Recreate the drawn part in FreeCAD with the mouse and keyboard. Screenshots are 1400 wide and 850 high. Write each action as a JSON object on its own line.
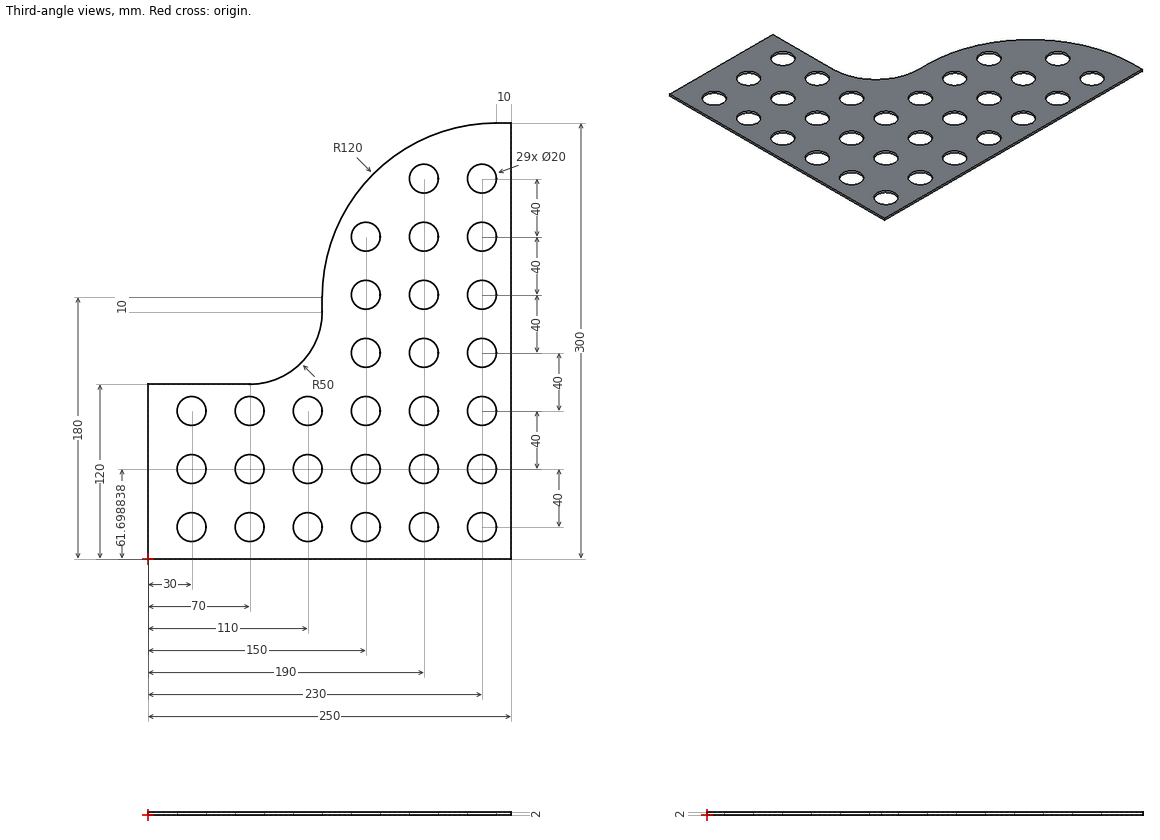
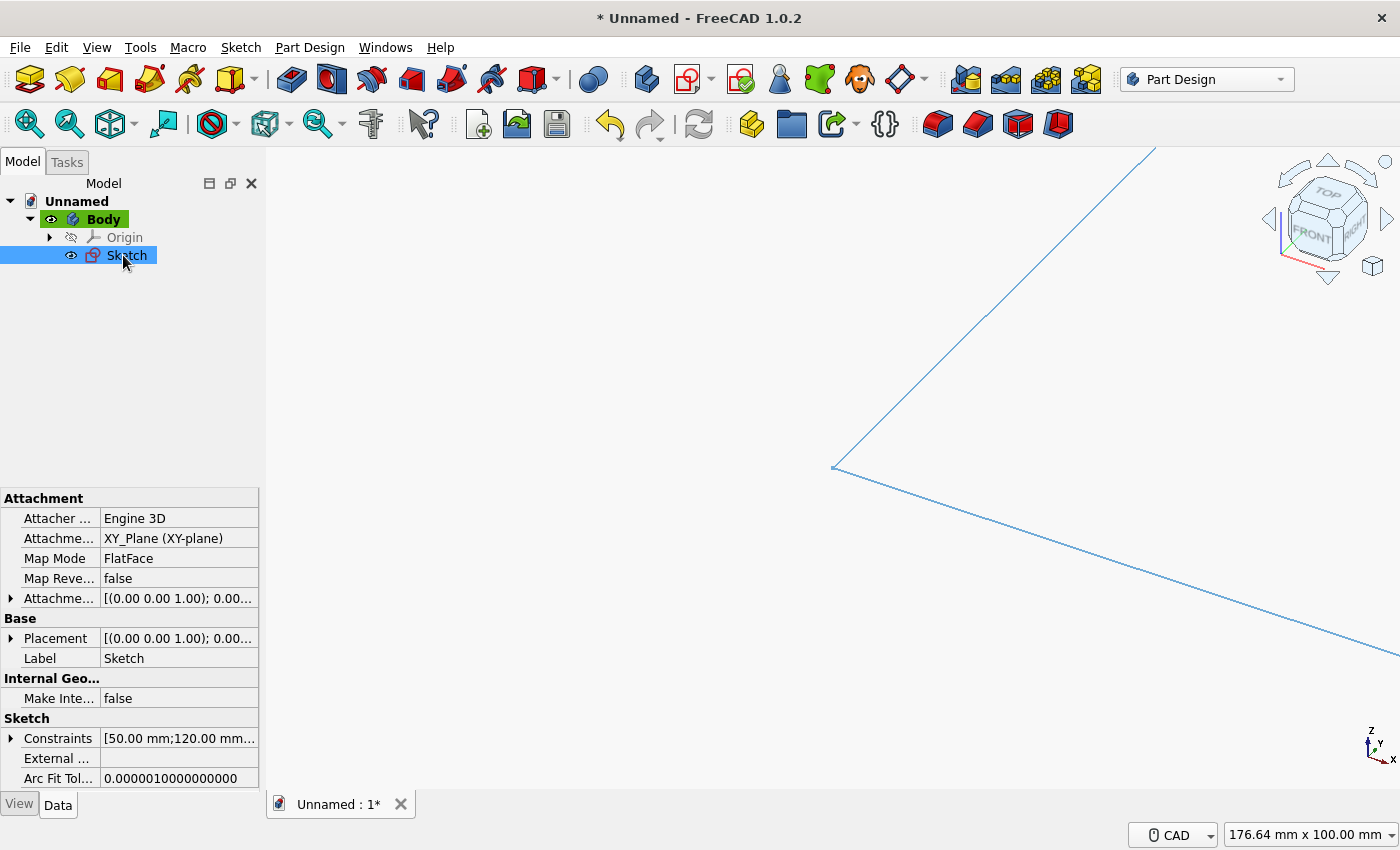
{"action": "left_click", "coordinate": [30, 80]}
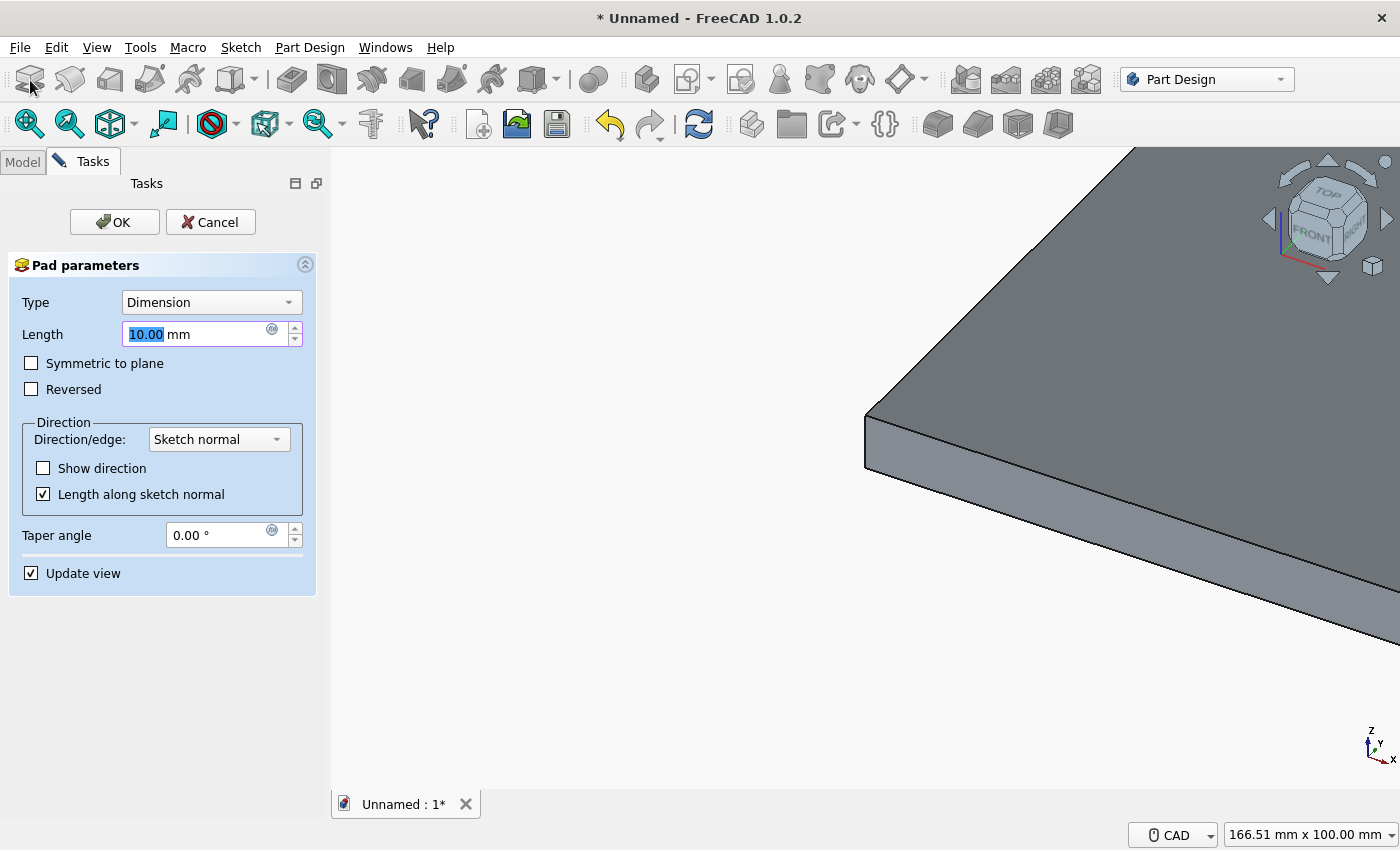
{"action": "type", "text": "2"}
{"action": "key", "text": "Tab"}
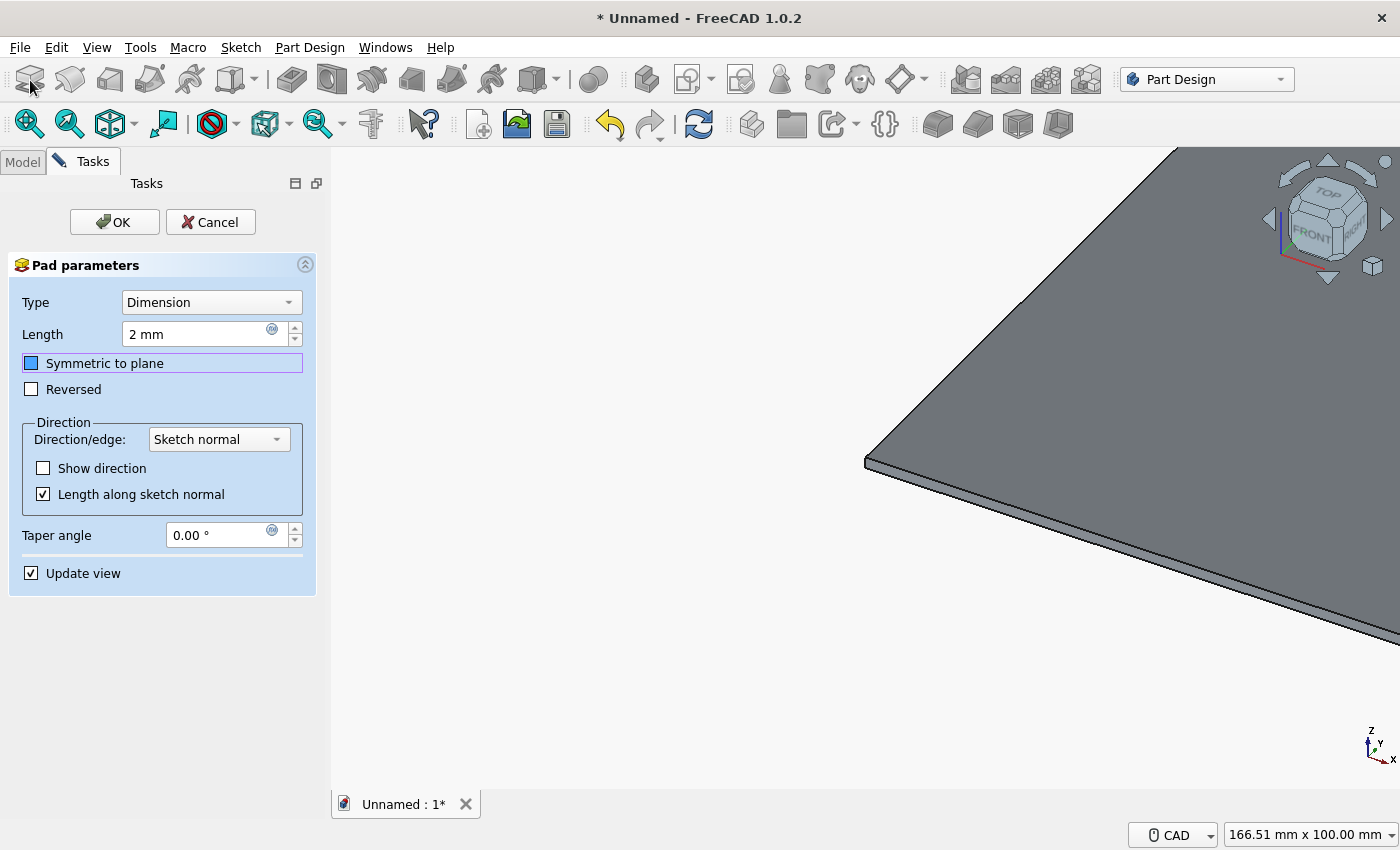
{"action": "left_click", "coordinate": [115, 222]}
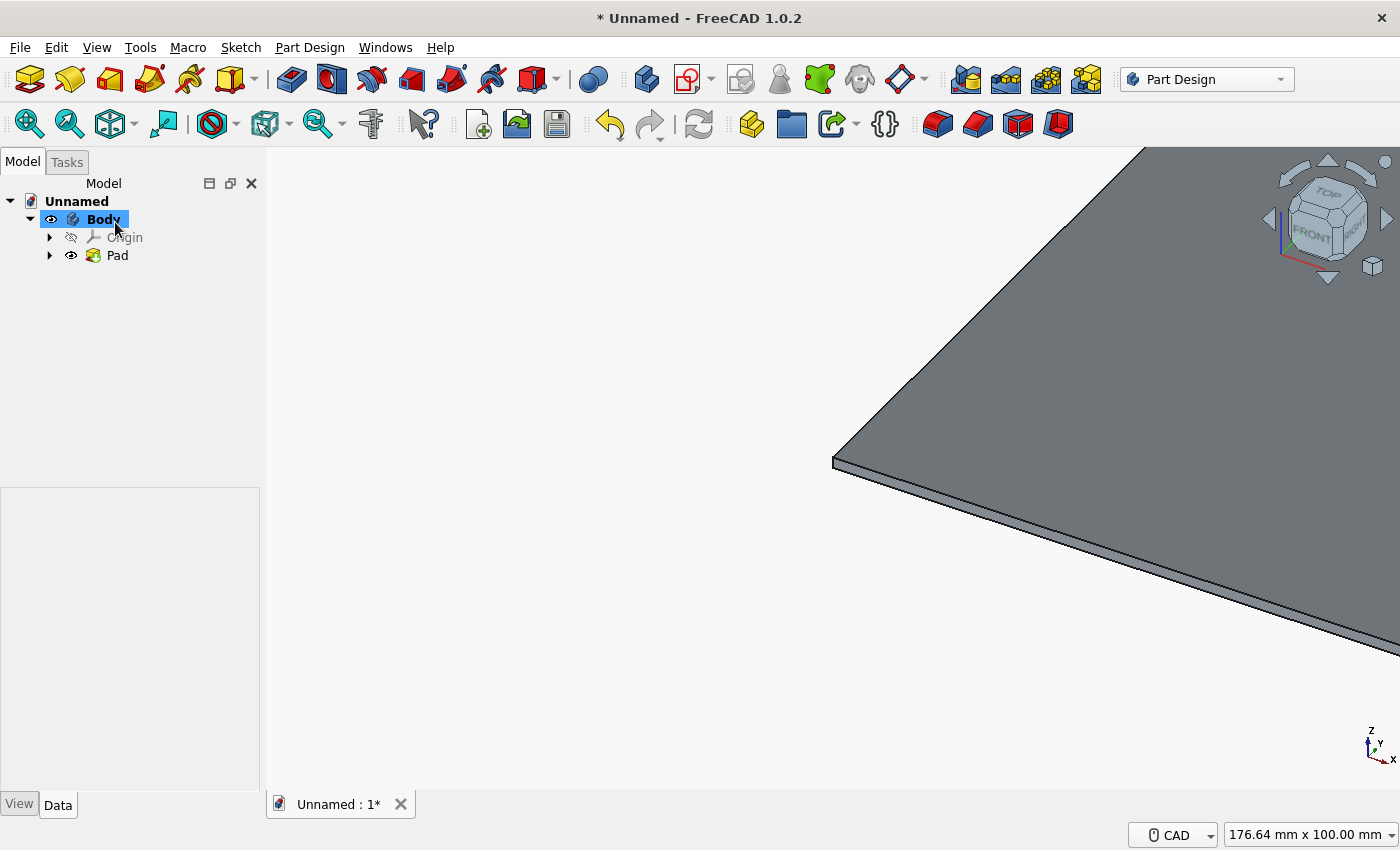
{"action": "key", "text": "v f"}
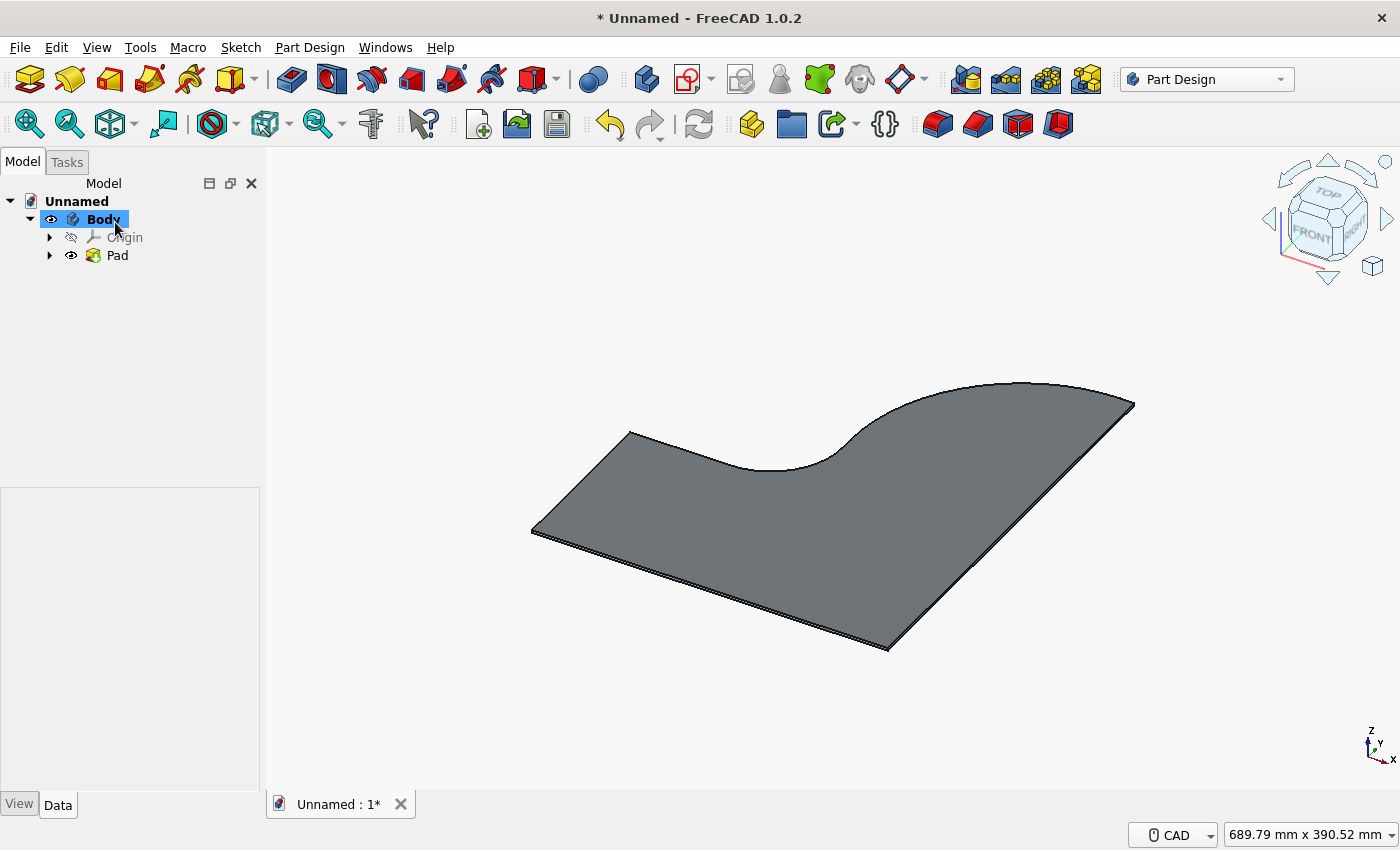
{"action": "left_click", "coordinate": [813, 552]}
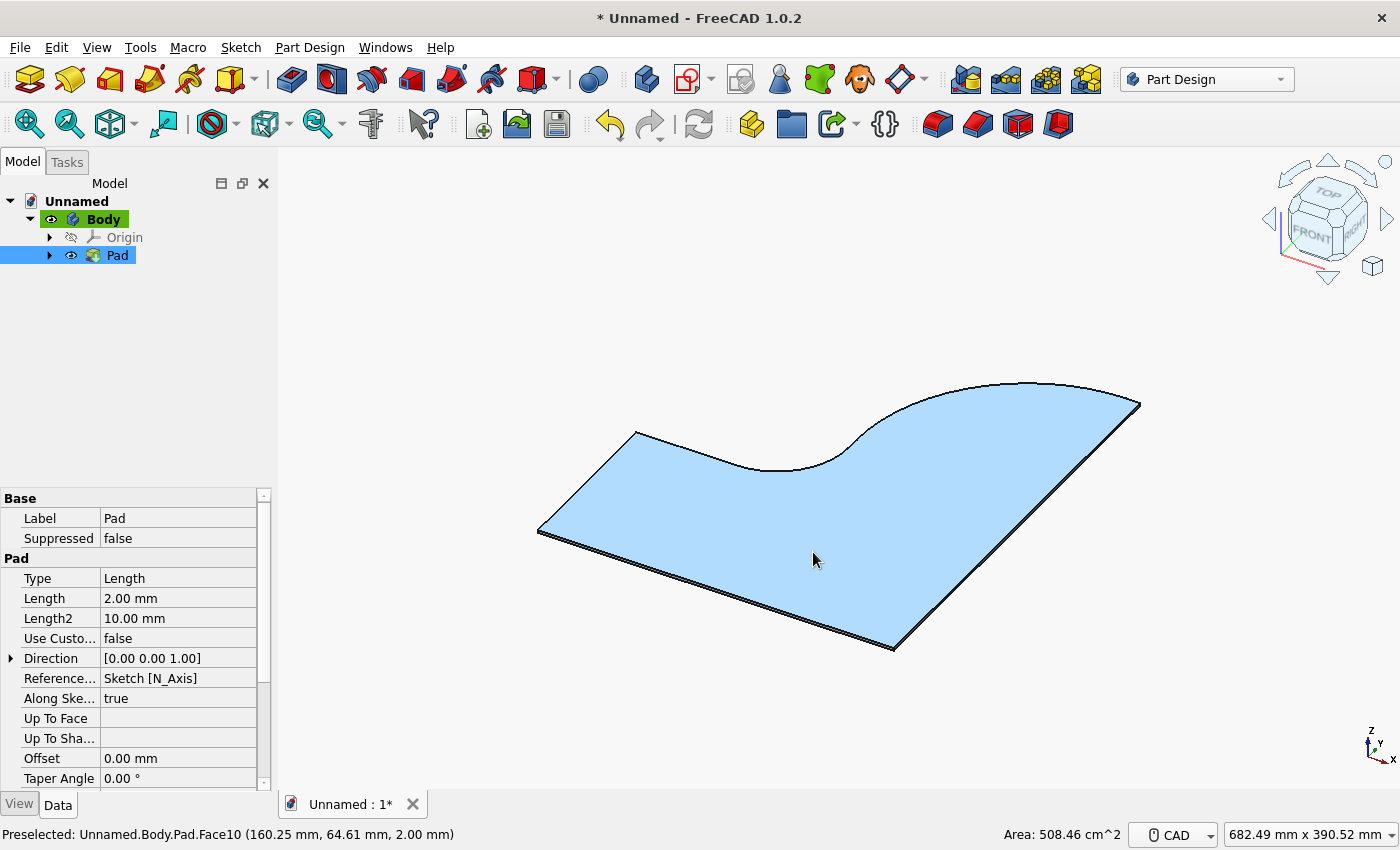
{"action": "left_click", "coordinate": [688, 80]}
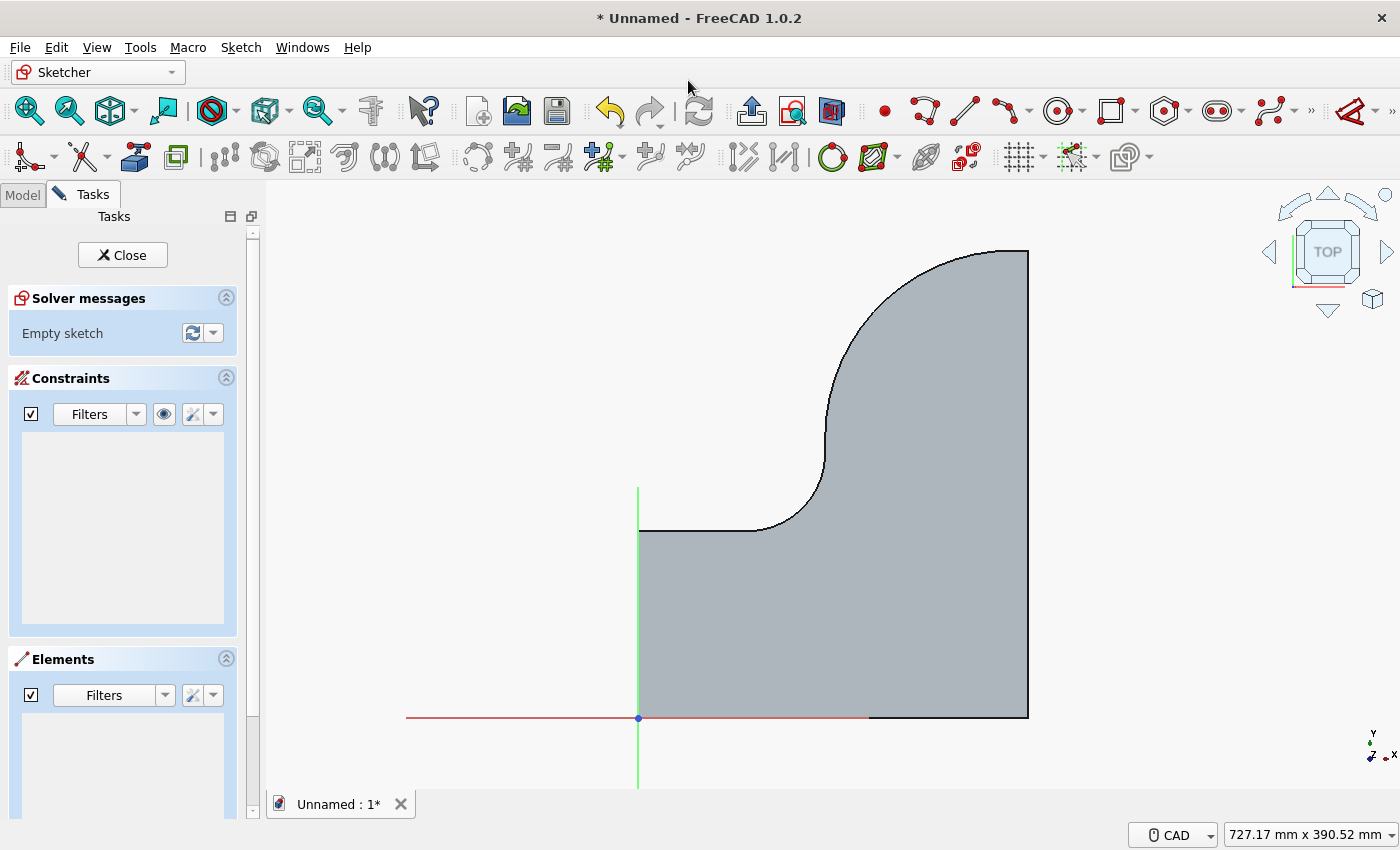
{"action": "left_click", "coordinate": [1058, 112]}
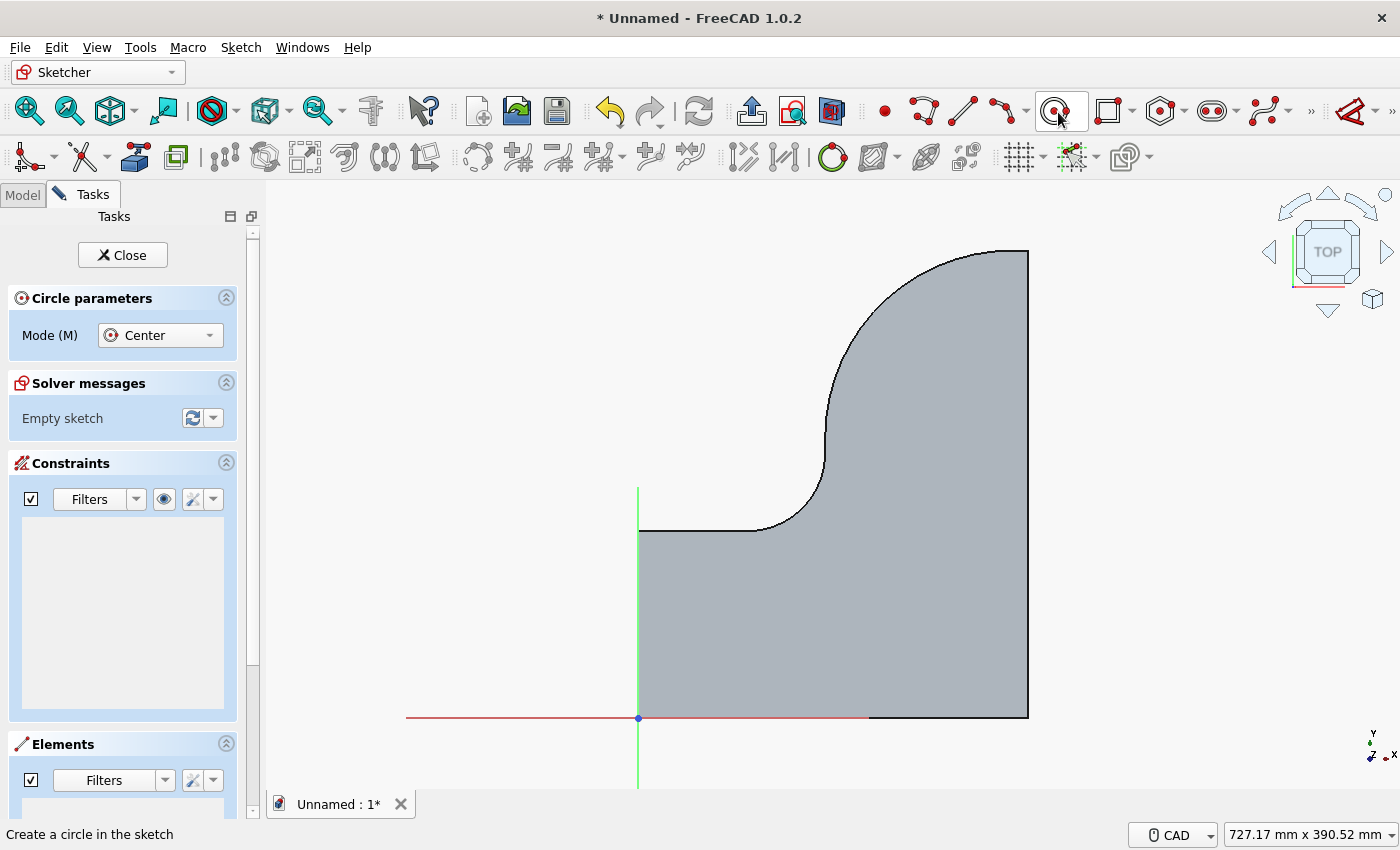
{"action": "scroll", "coordinate": [997, 310], "scroll_direction": "up", "scroll_amount": 2}